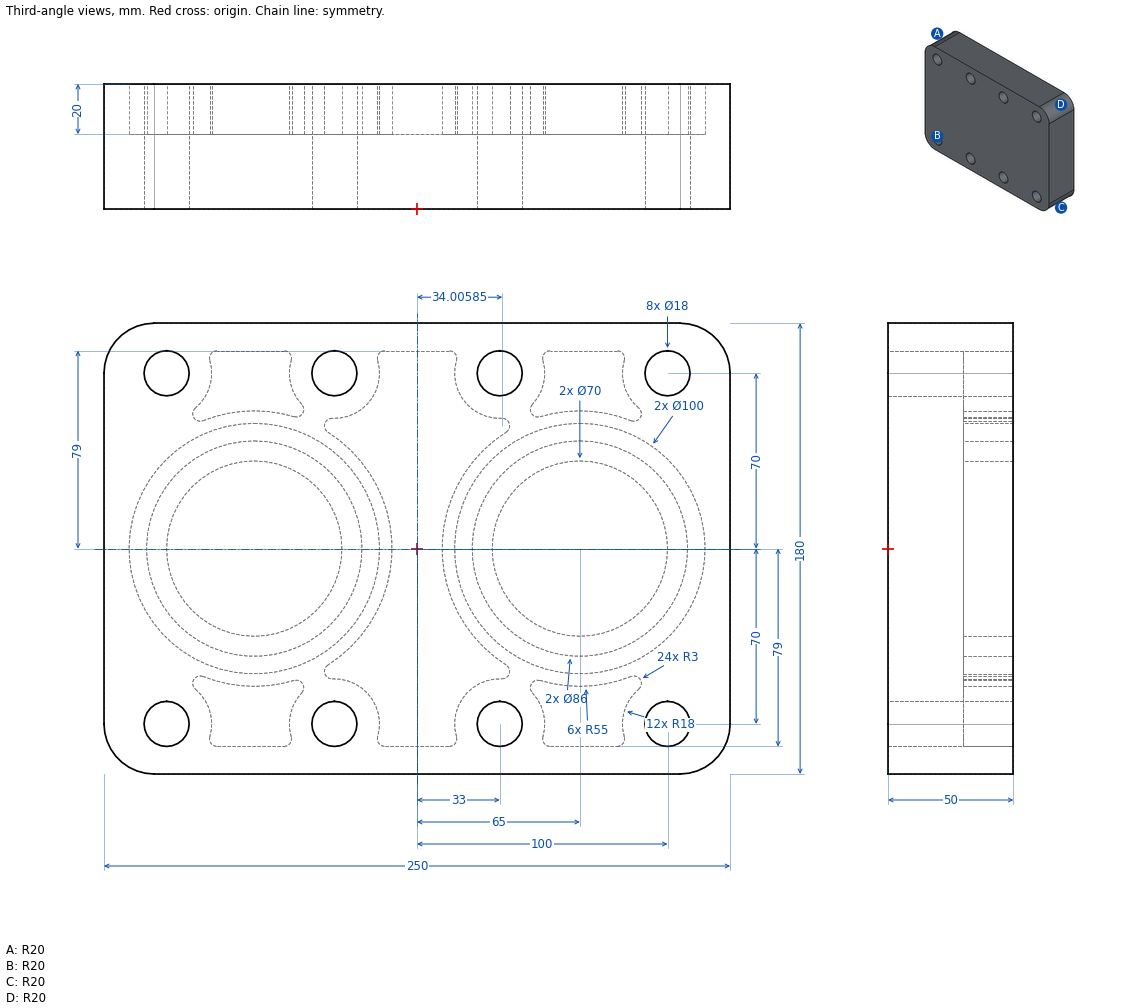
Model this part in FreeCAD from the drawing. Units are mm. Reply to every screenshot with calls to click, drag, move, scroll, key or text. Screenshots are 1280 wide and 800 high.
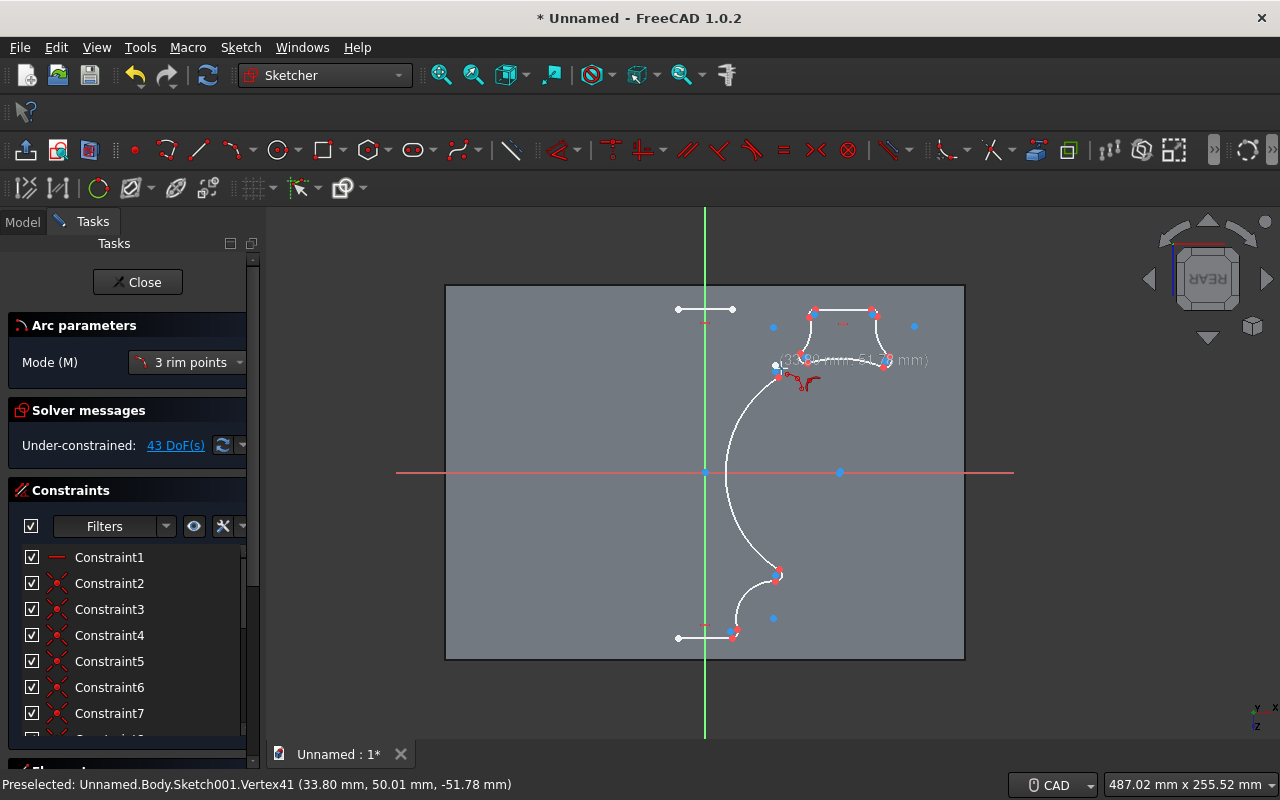
scroll(738, 316, up, 3)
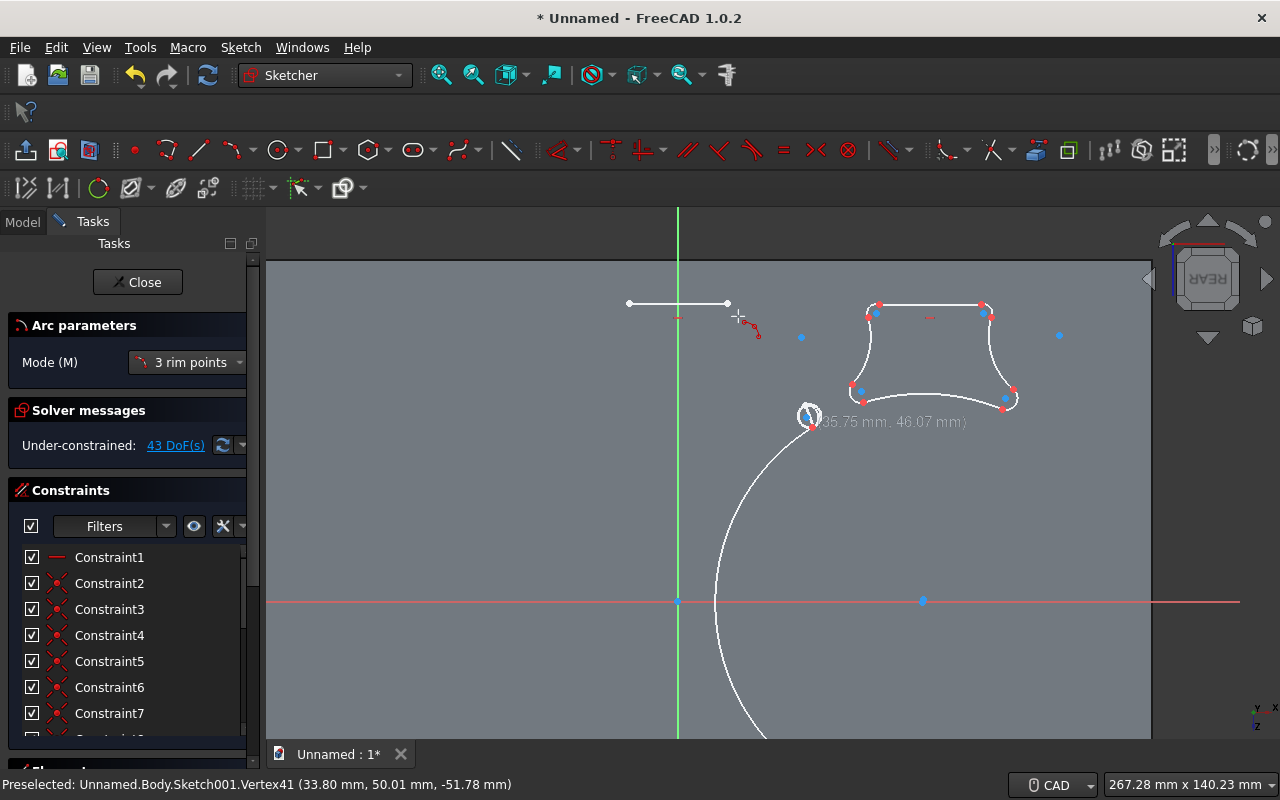
click(737, 317)
click(749, 378)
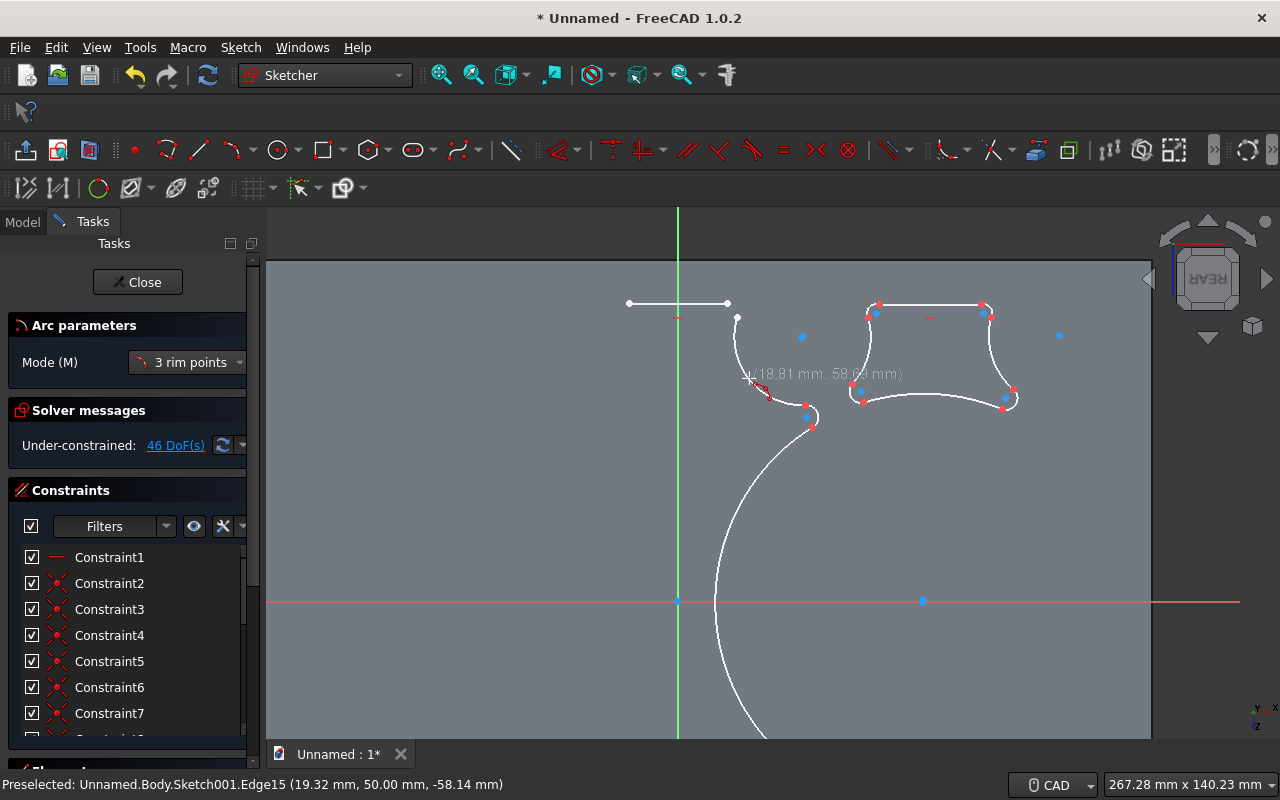
click(737, 318)
click(727, 304)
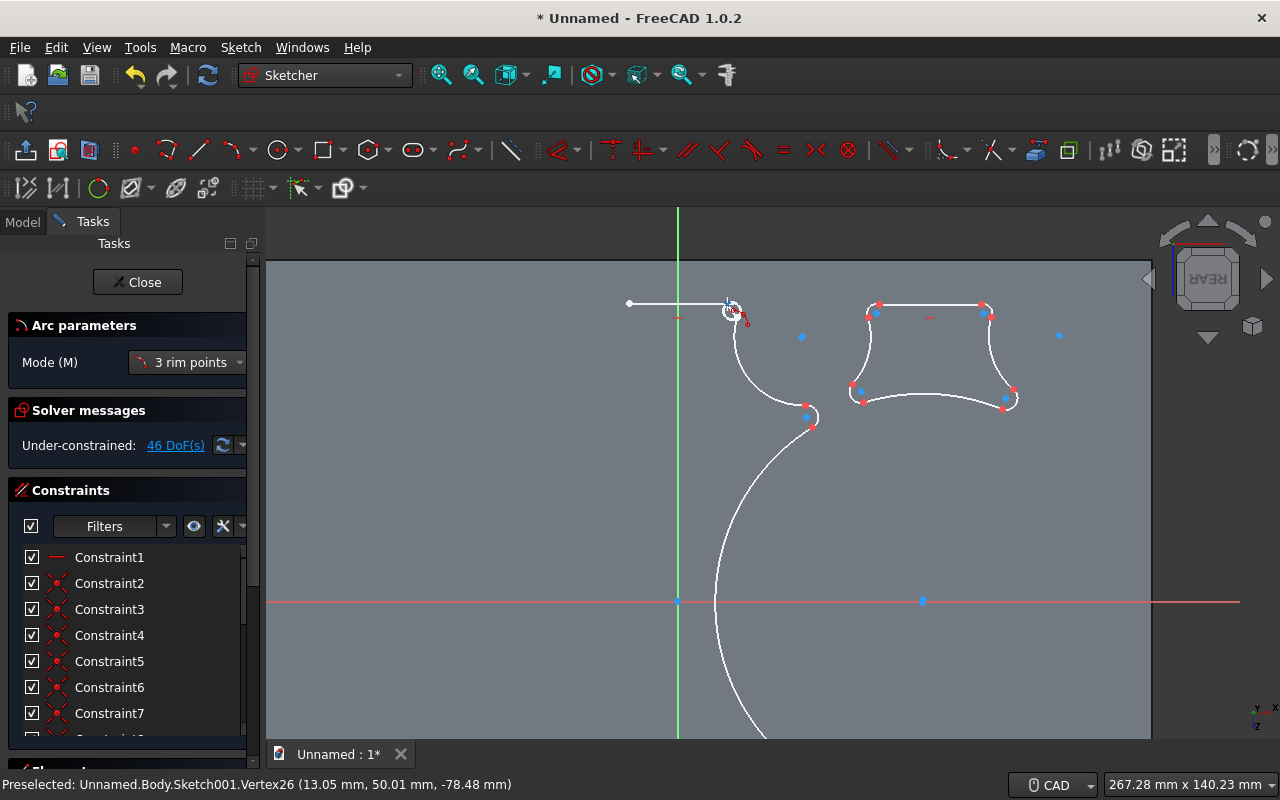
scroll(736, 307, up, 7)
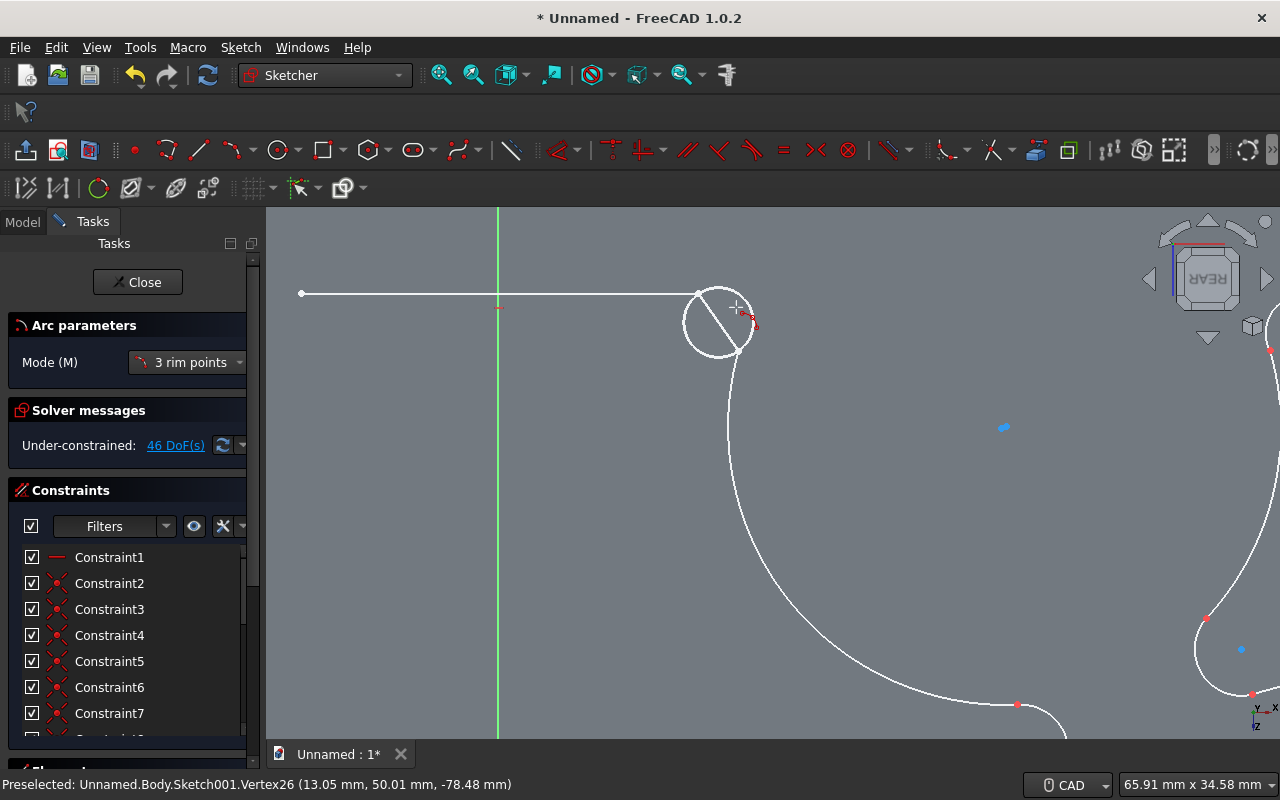
click(733, 305)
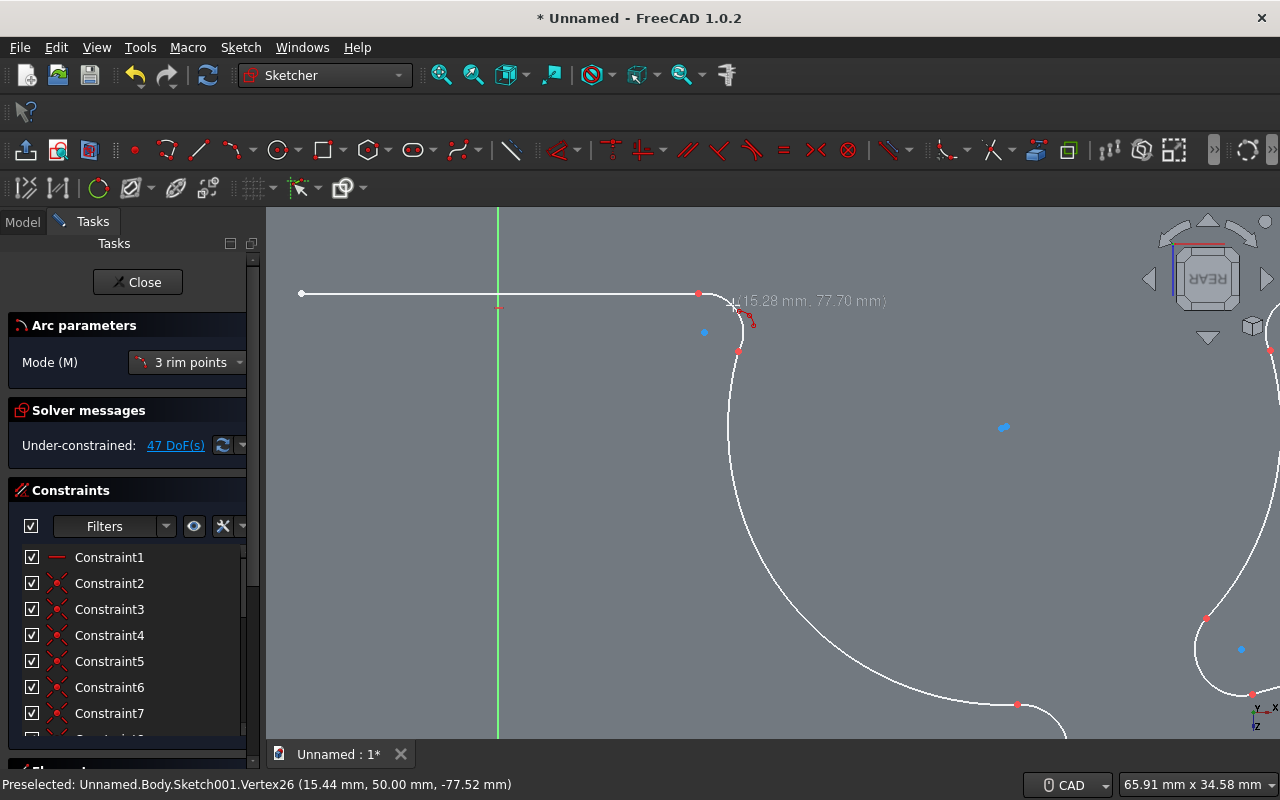
scroll(737, 312, down, 10)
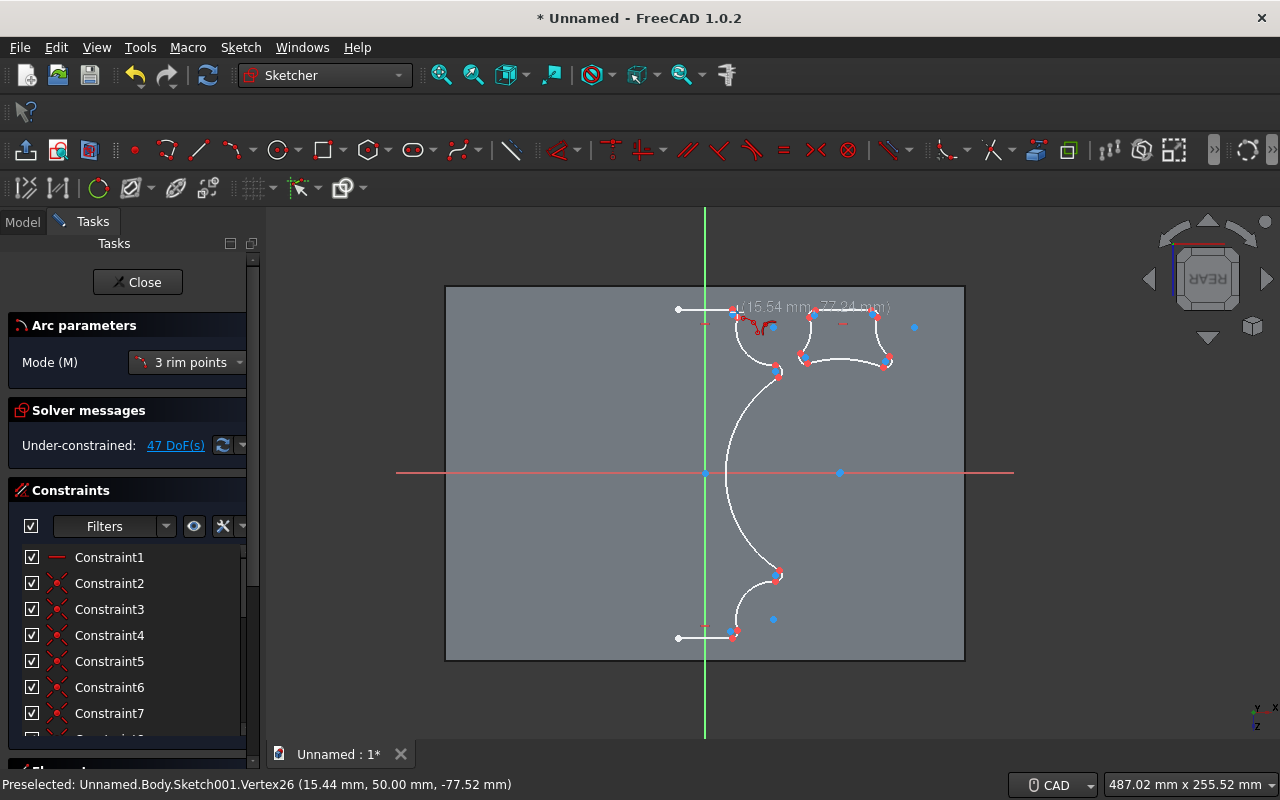
click(678, 310)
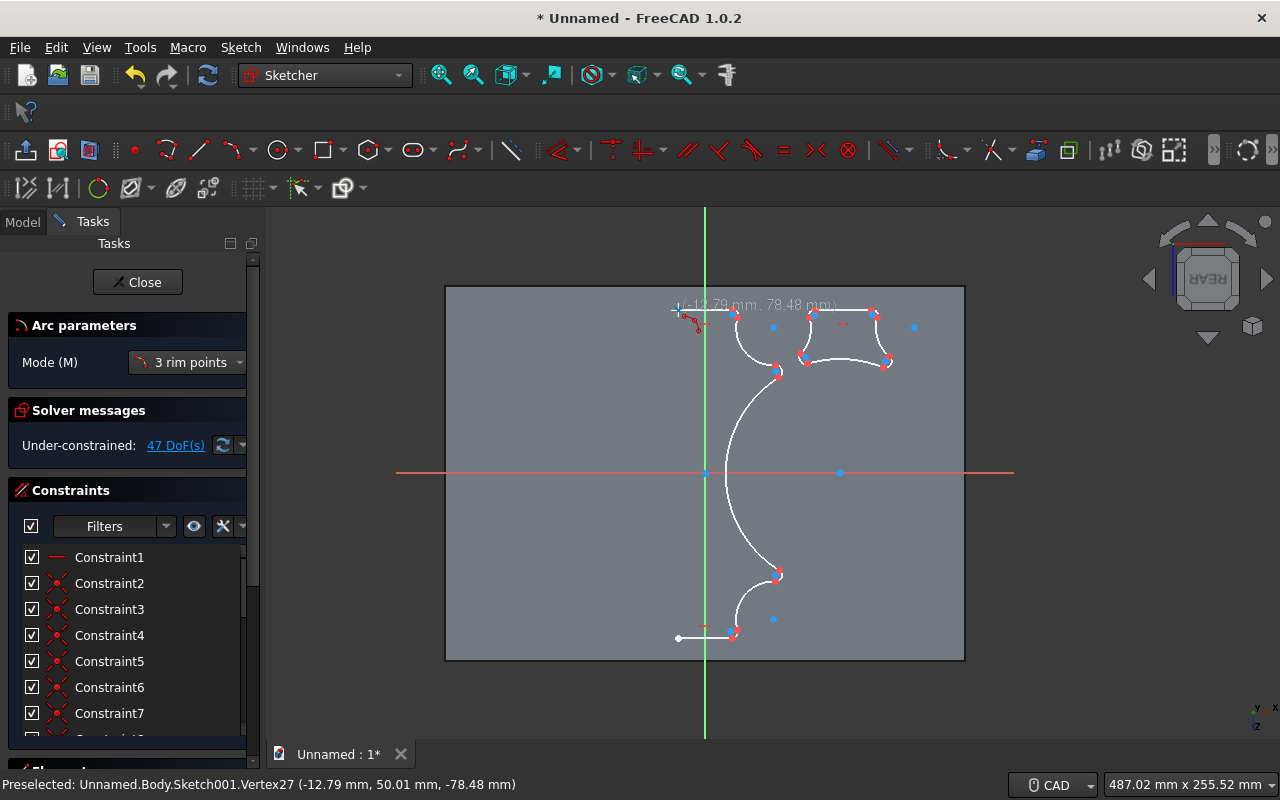
scroll(672, 317, up, 3)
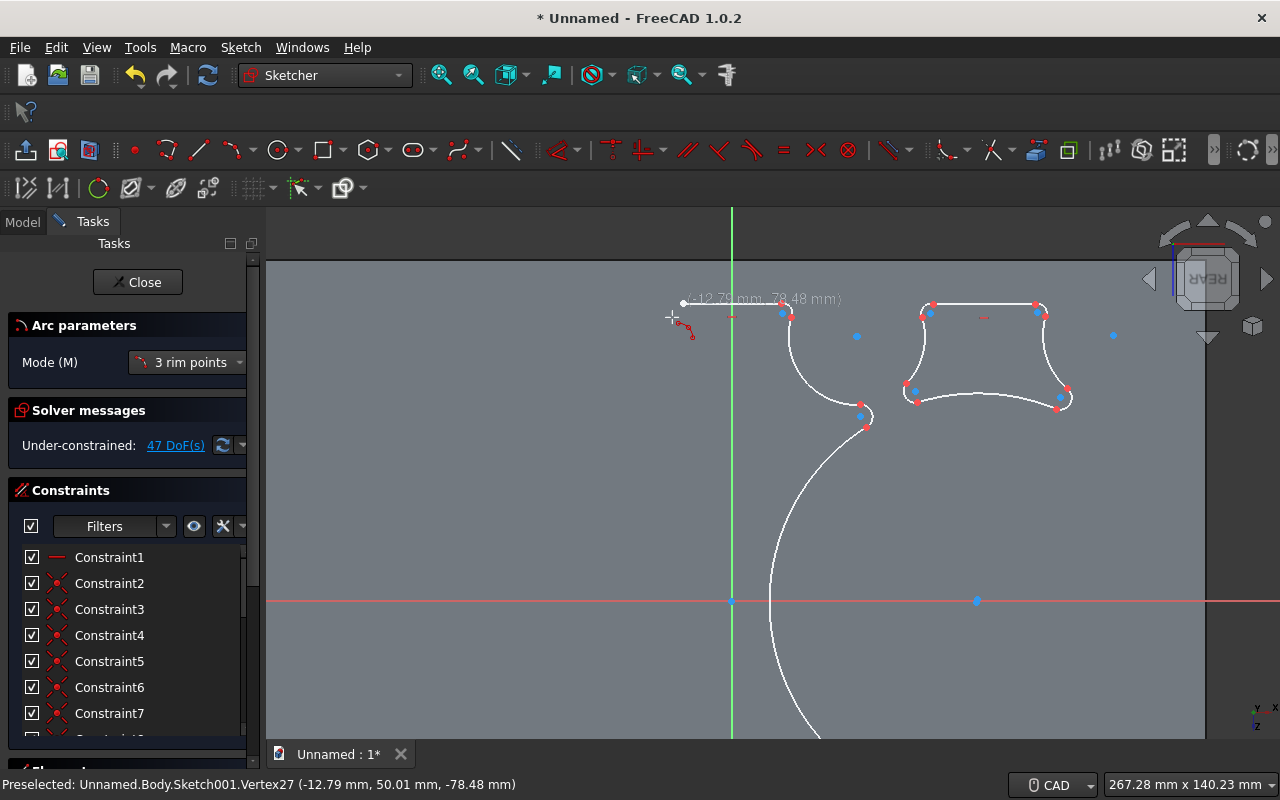
click(672, 316)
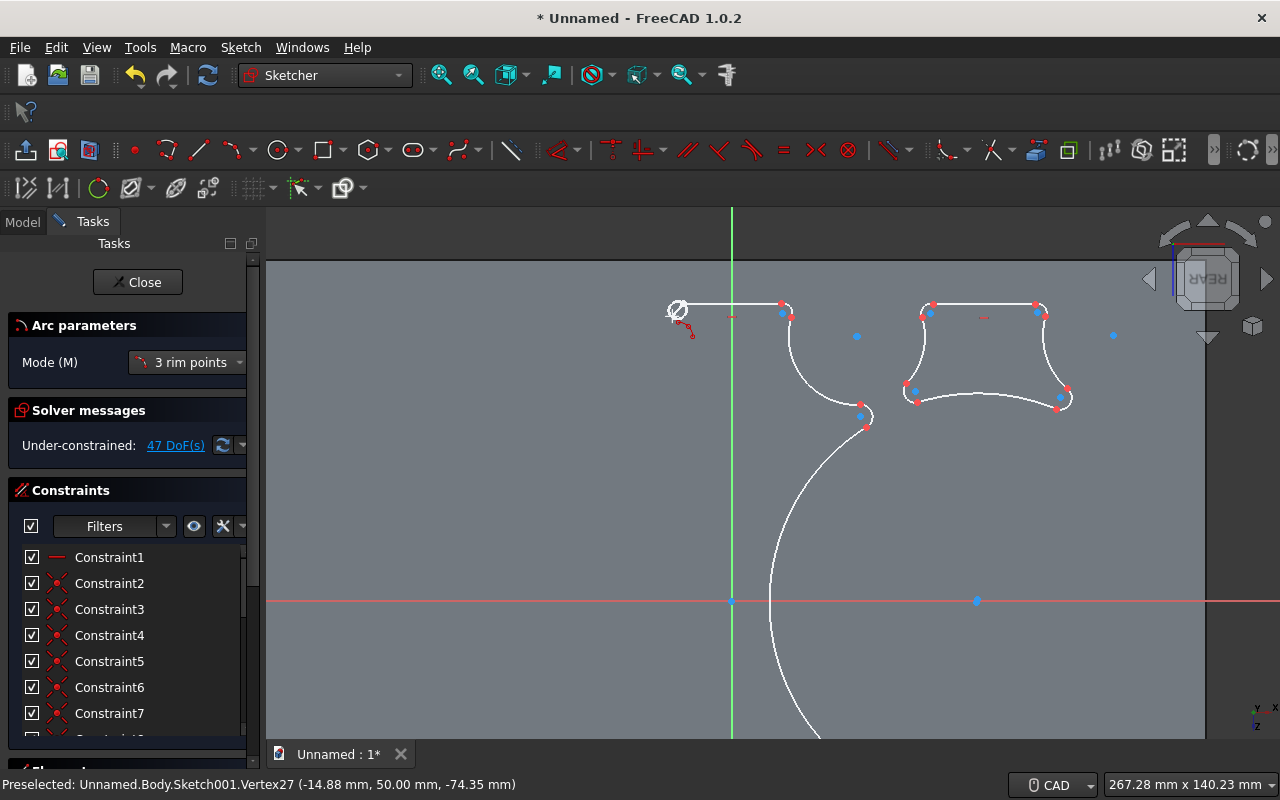
scroll(674, 306, up, 7)